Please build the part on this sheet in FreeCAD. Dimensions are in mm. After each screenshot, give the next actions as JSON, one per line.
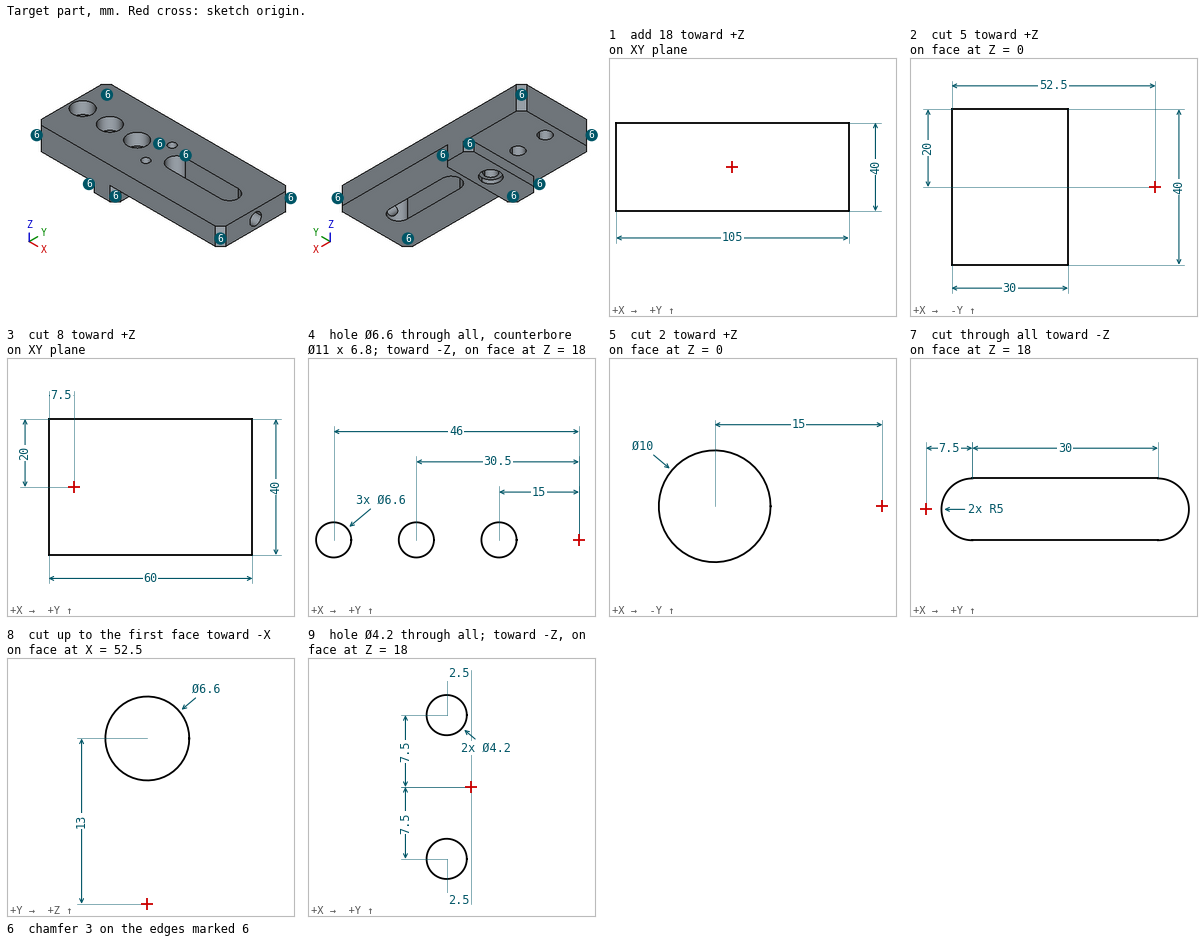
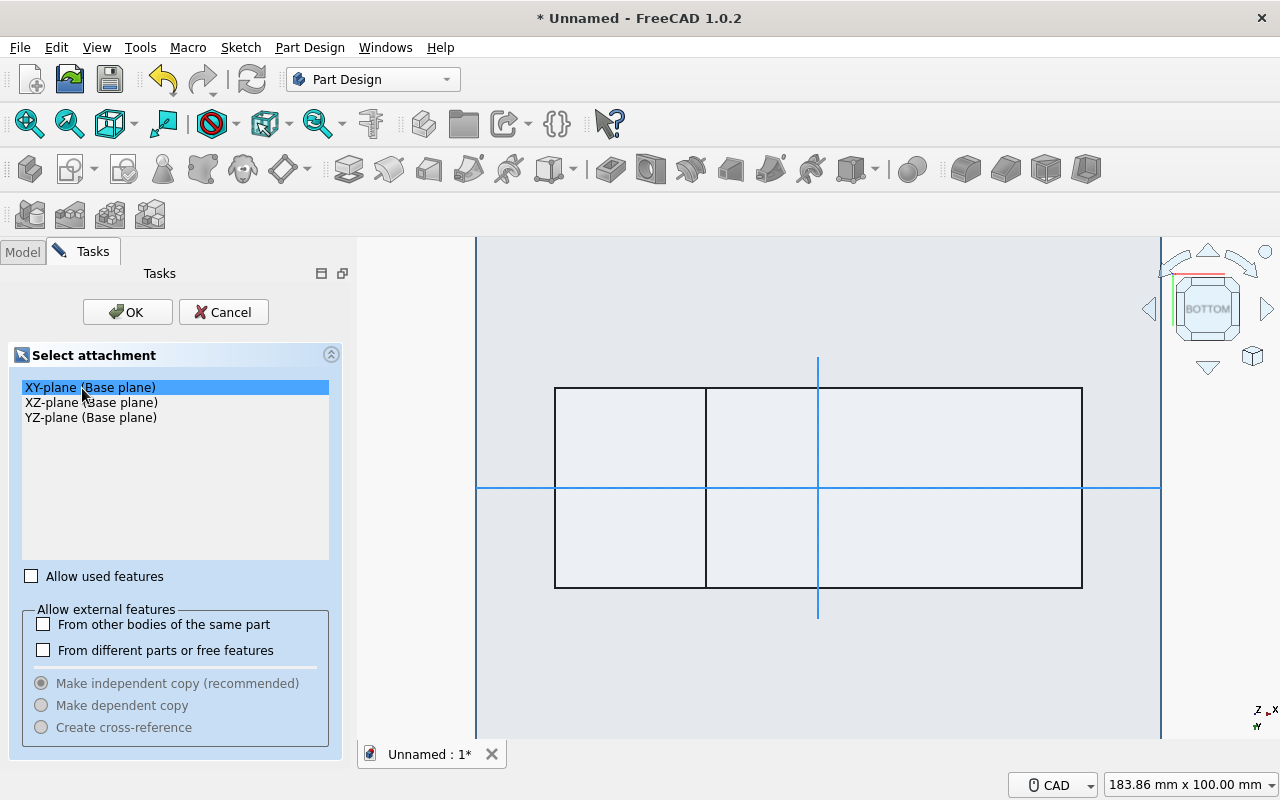
{"action": "left_click", "coordinate": [128, 312]}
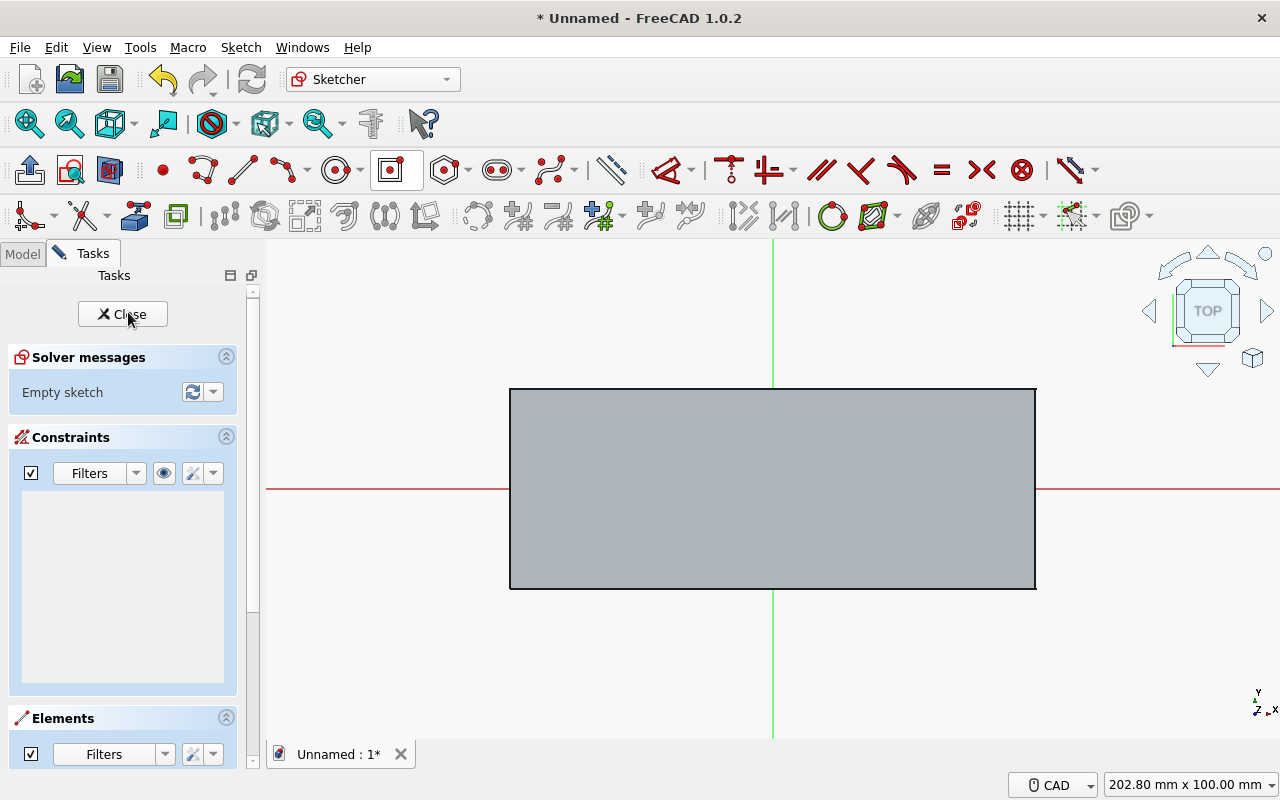
{"action": "left_click", "coordinate": [110, 170]}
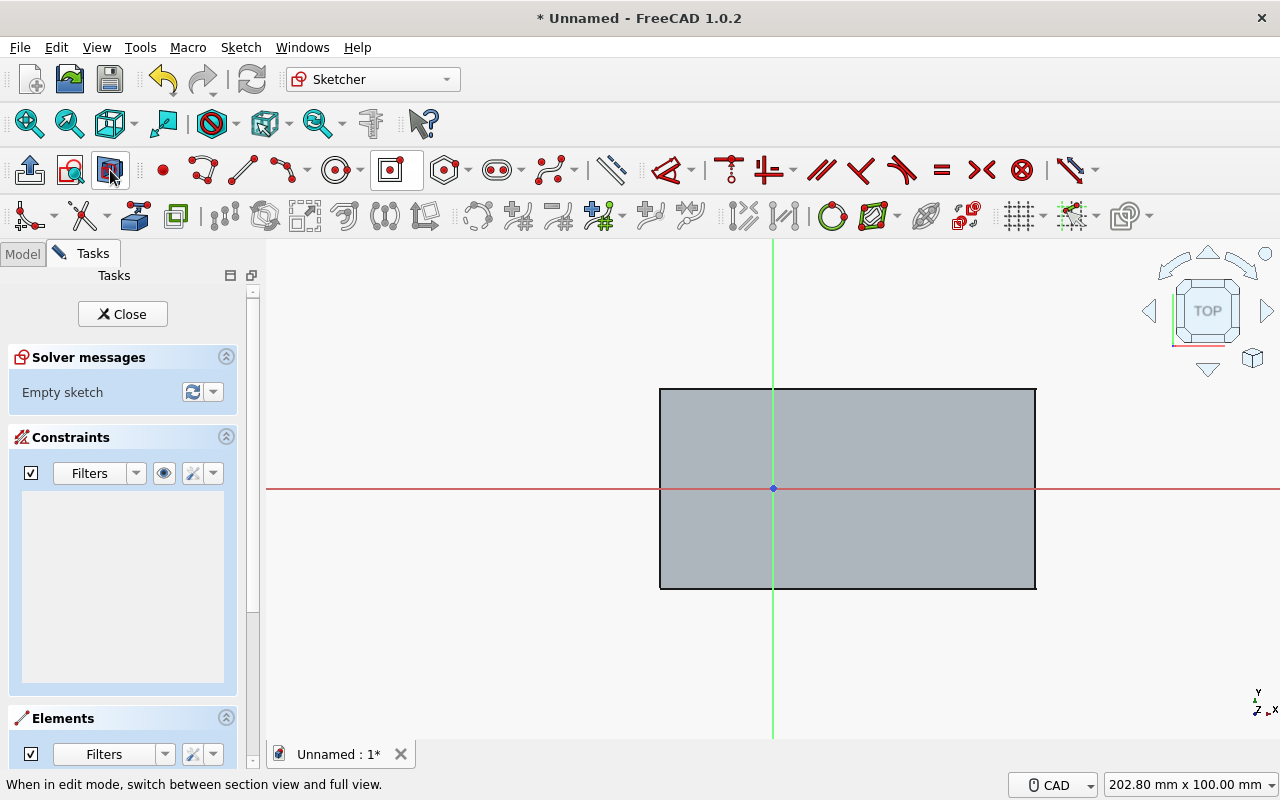
{"action": "scroll", "coordinate": [1115, 489], "scroll_direction": "up", "scroll_amount": 2}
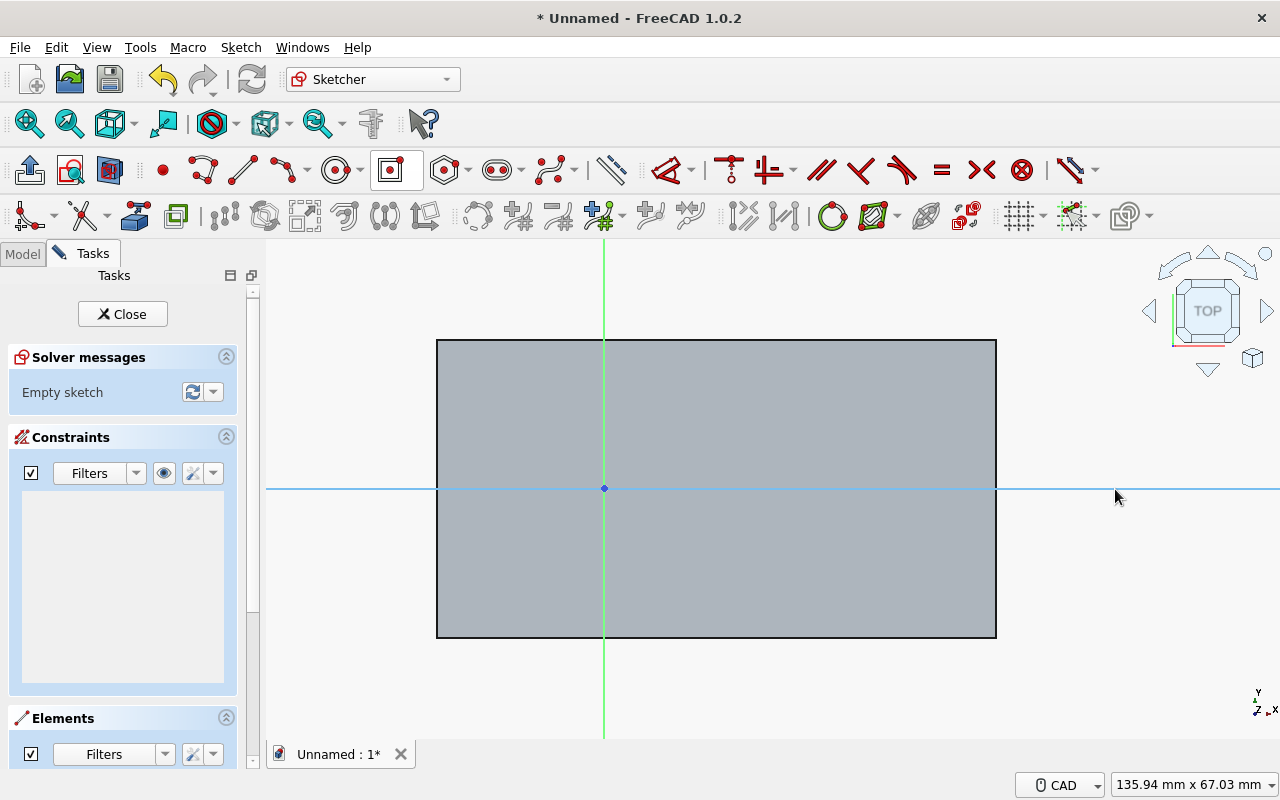
{"action": "key", "text": "g r"}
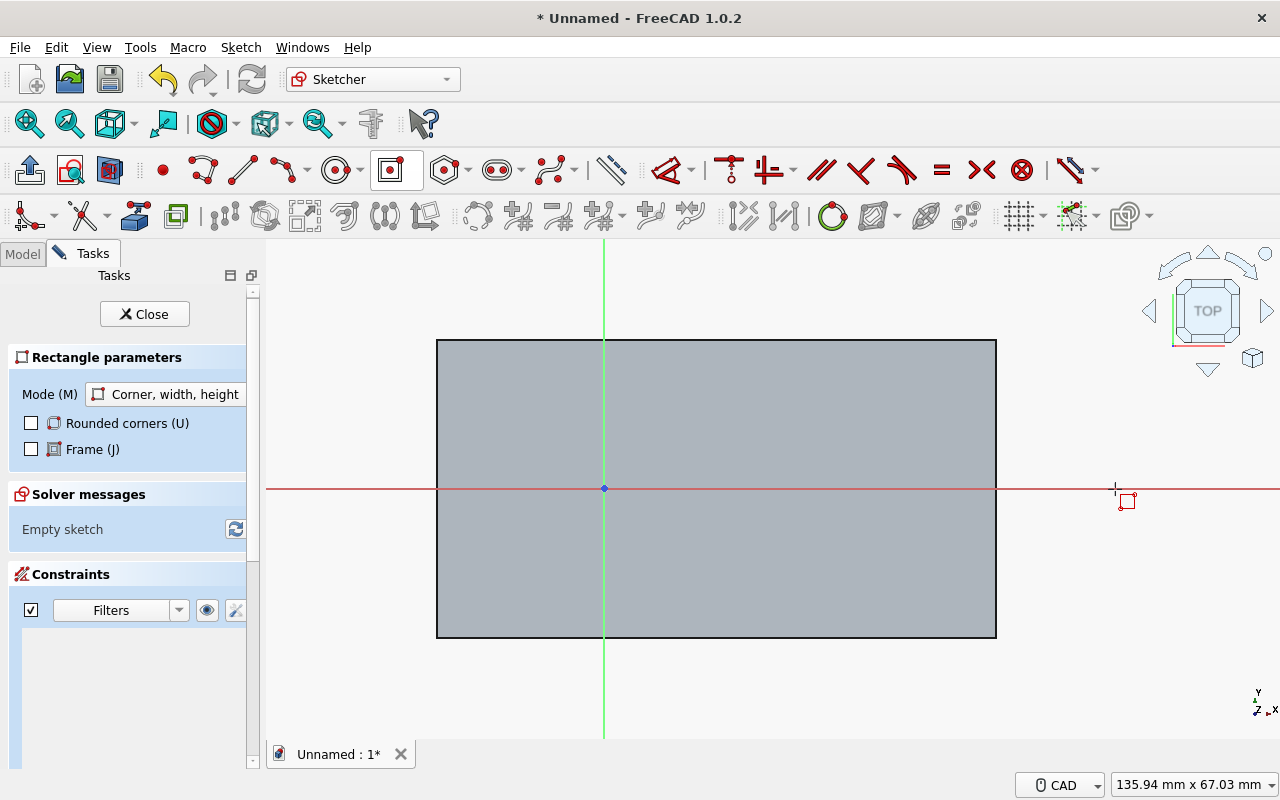
{"action": "left_click", "coordinate": [548, 340]}
{"action": "mouse_move", "coordinate": [996, 638]}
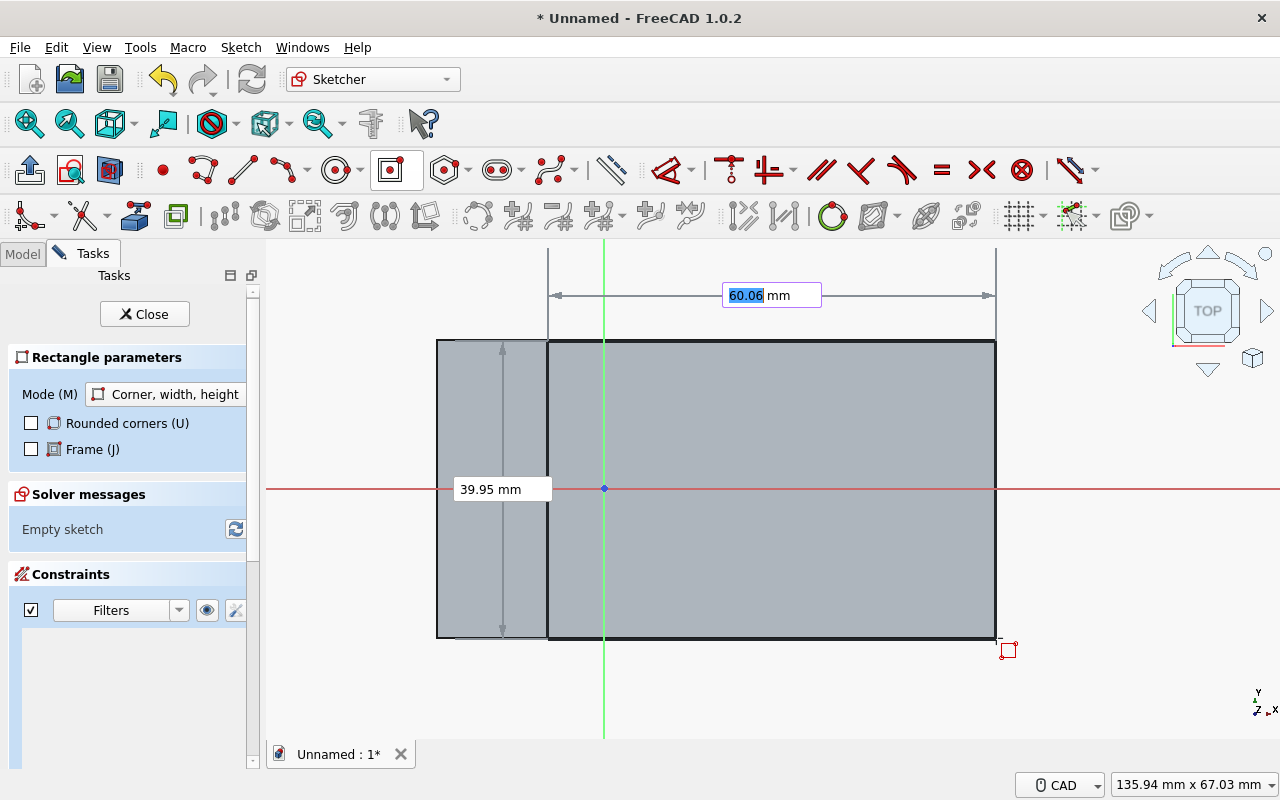
{"action": "type", "text": "60"}
{"action": "key", "text": "Tab"}
{"action": "type", "text": "40"}
{"action": "key", "text": "Return"}
{"action": "key", "text": "Escape"}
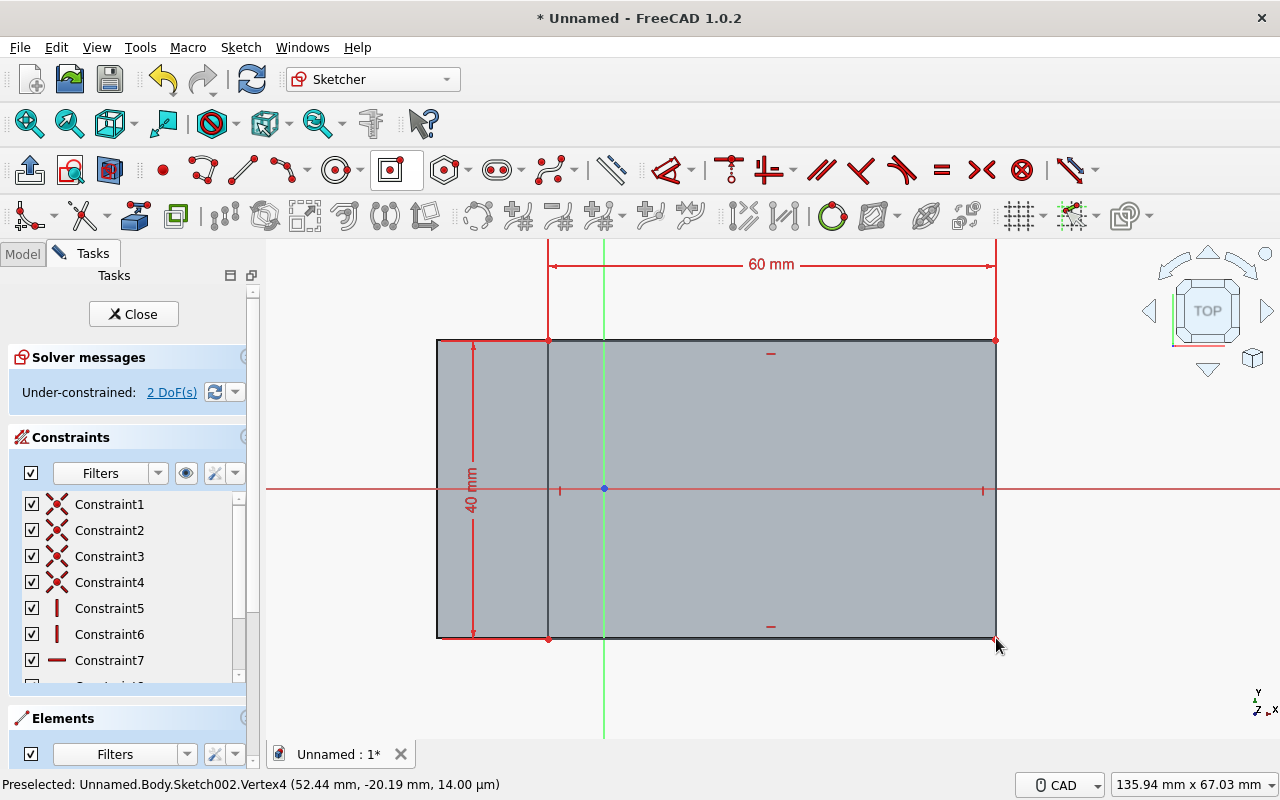
{"action": "left_click", "coordinate": [666, 170]}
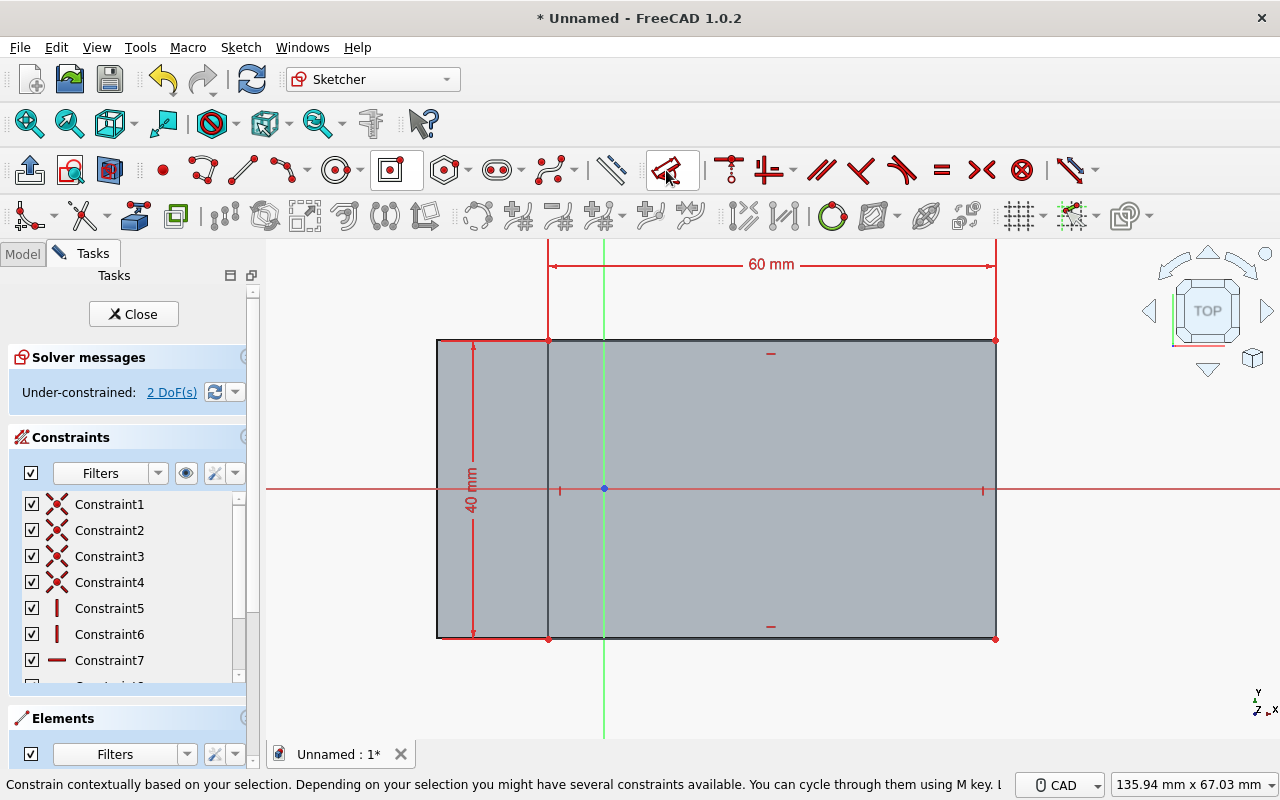
{"action": "left_click", "coordinate": [548, 341]}
{"action": "left_click", "coordinate": [514, 415]}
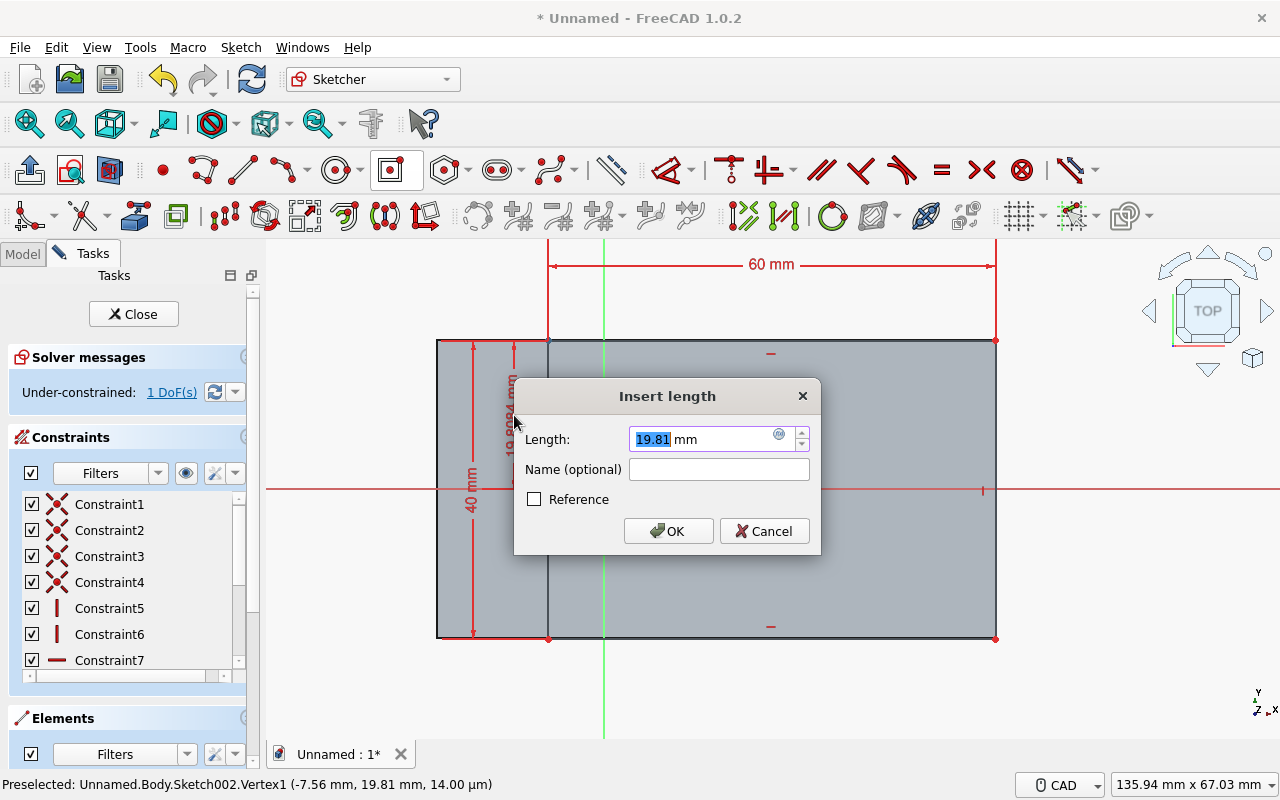
{"action": "type", "text": "20"}
{"action": "key", "text": "Return"}